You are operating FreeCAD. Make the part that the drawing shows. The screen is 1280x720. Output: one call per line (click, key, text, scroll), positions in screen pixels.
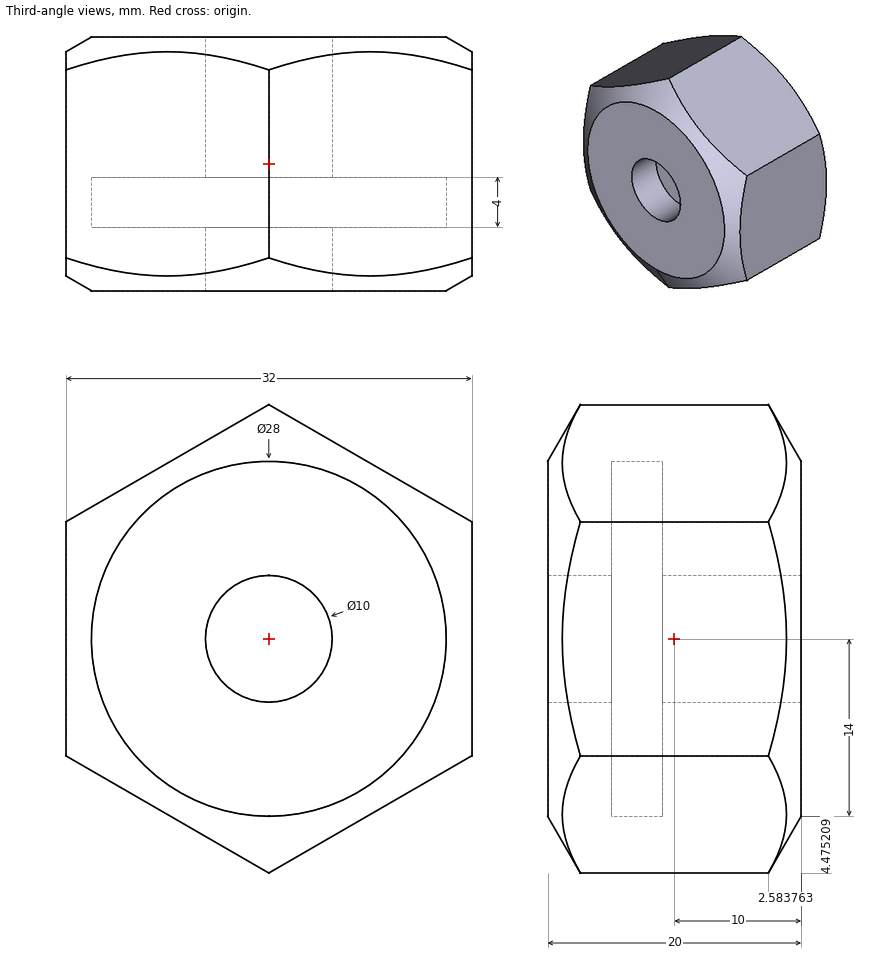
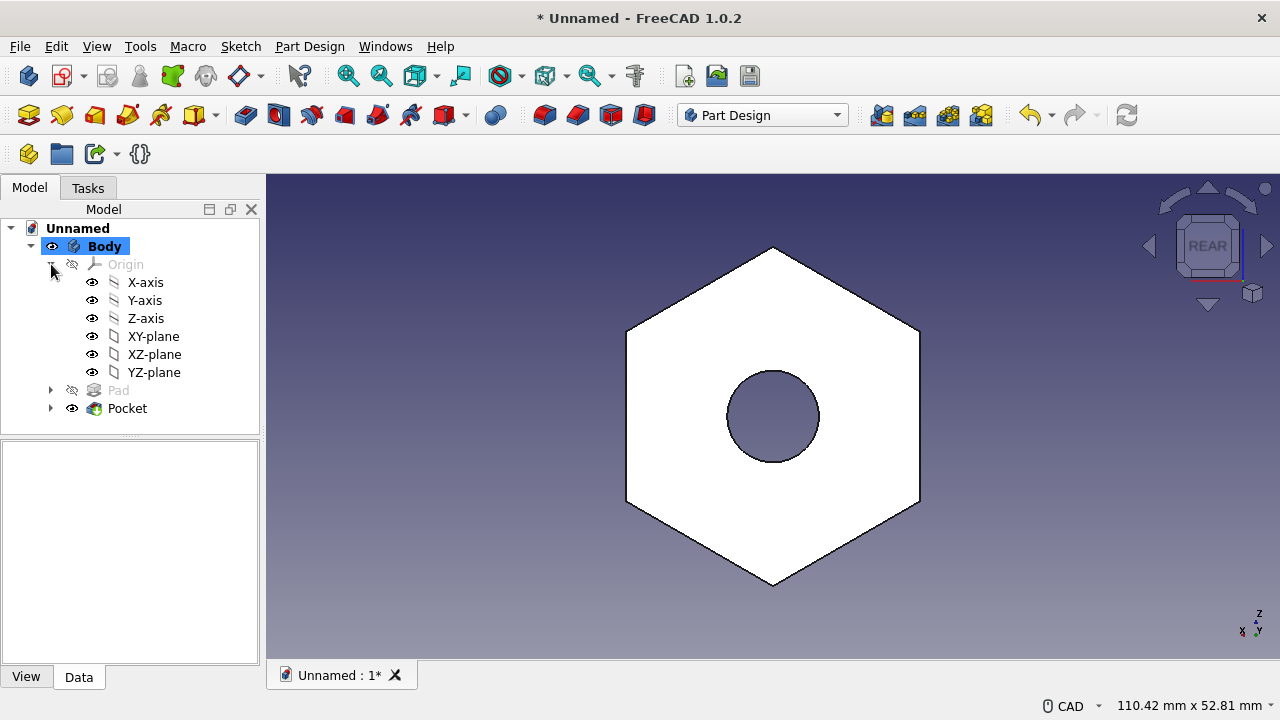
click(137, 354)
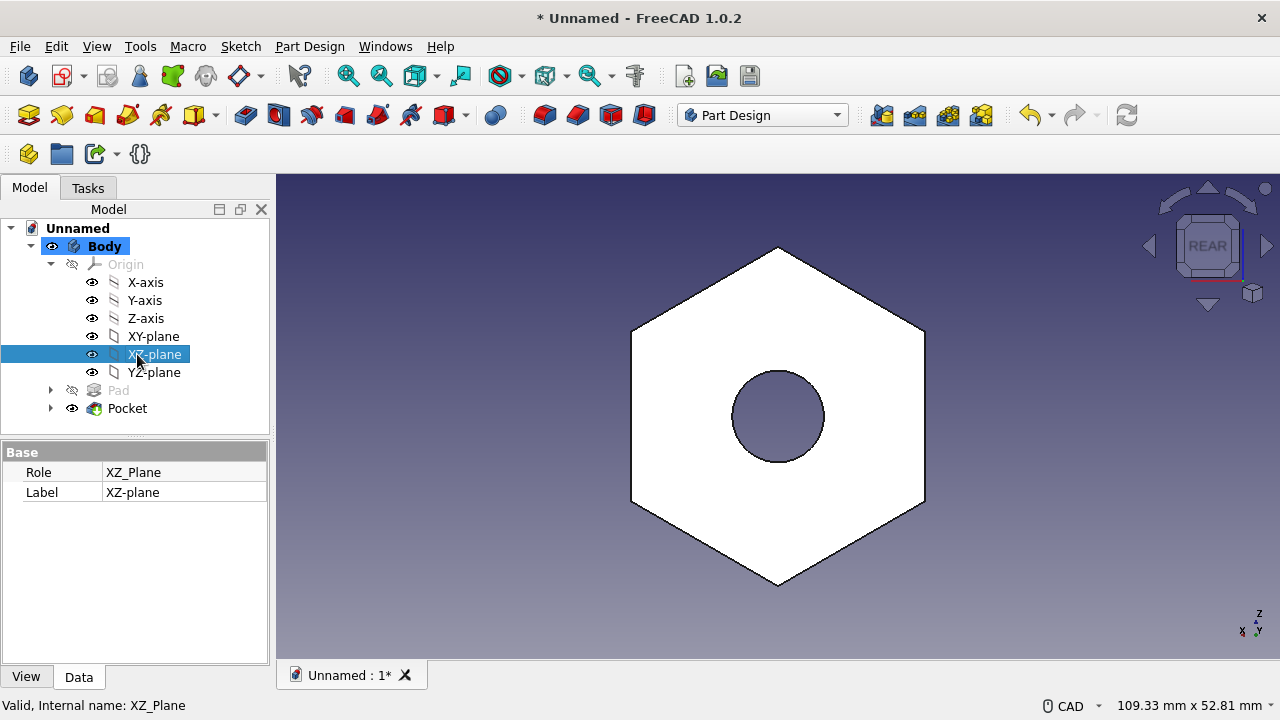
click(238, 76)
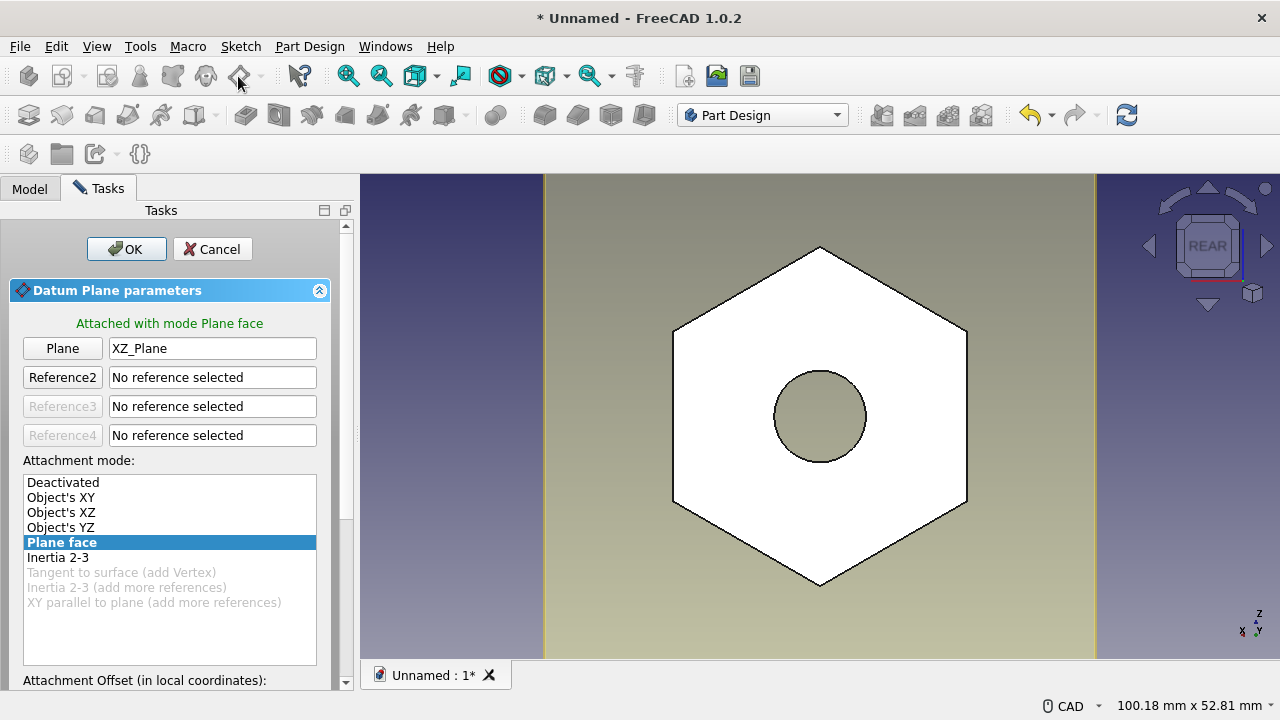
scroll(346, 455, down, 3)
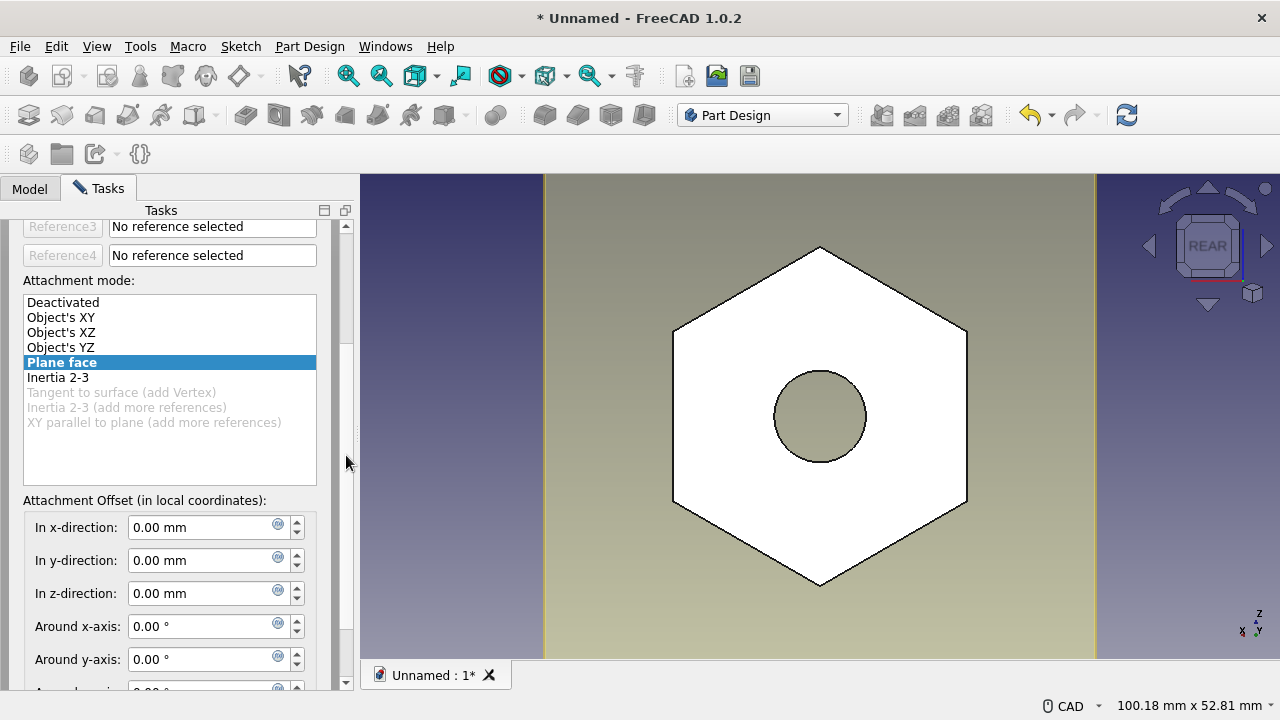
triple_click(210, 594)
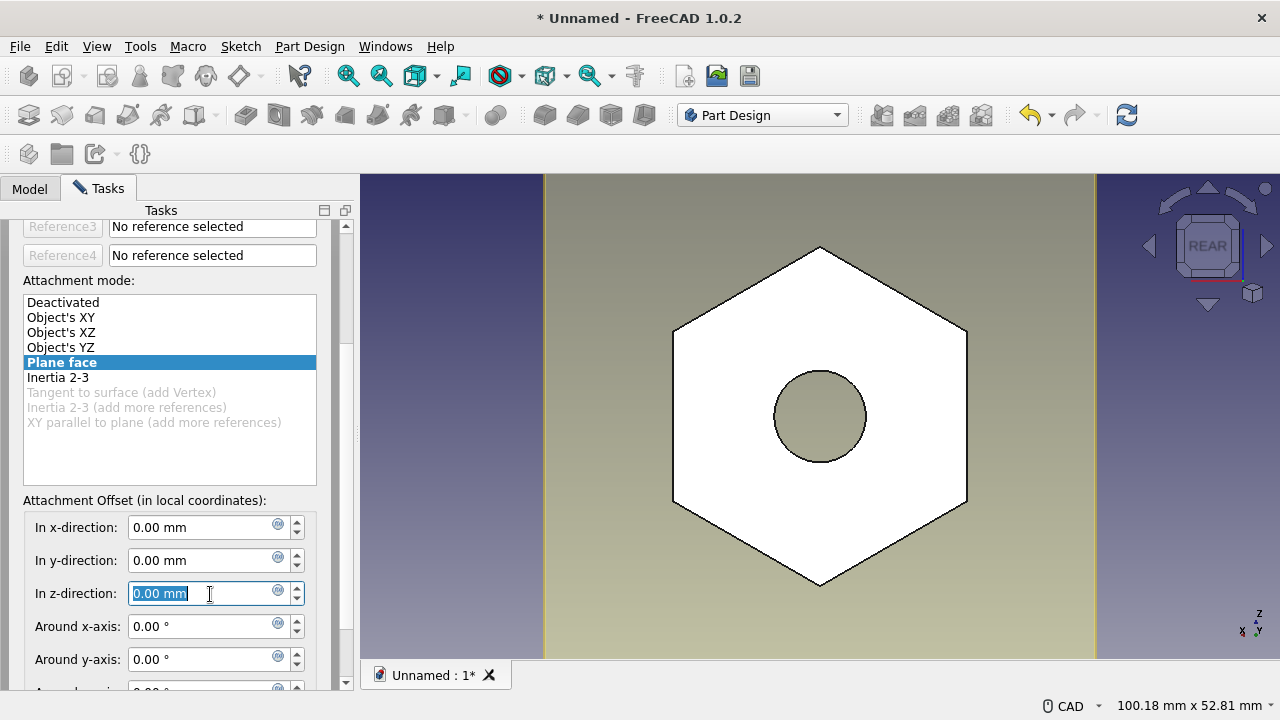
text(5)
key(Tab)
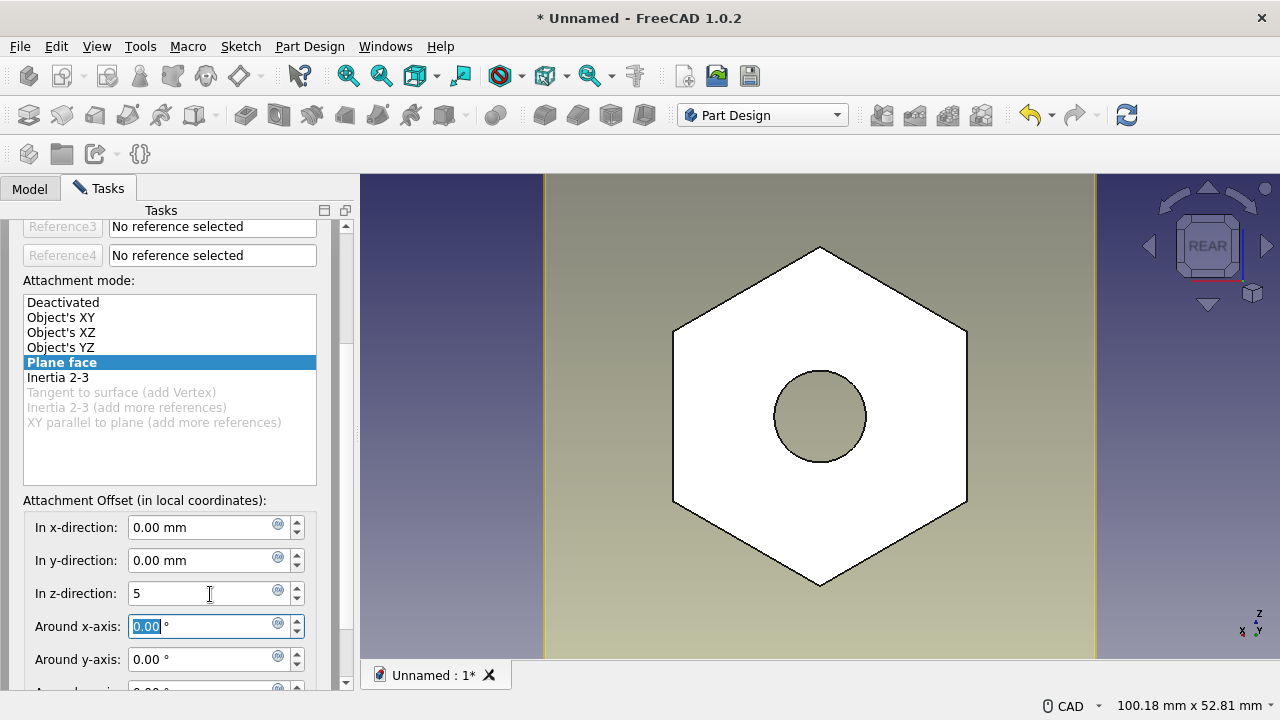
scroll(346, 455, up, 4)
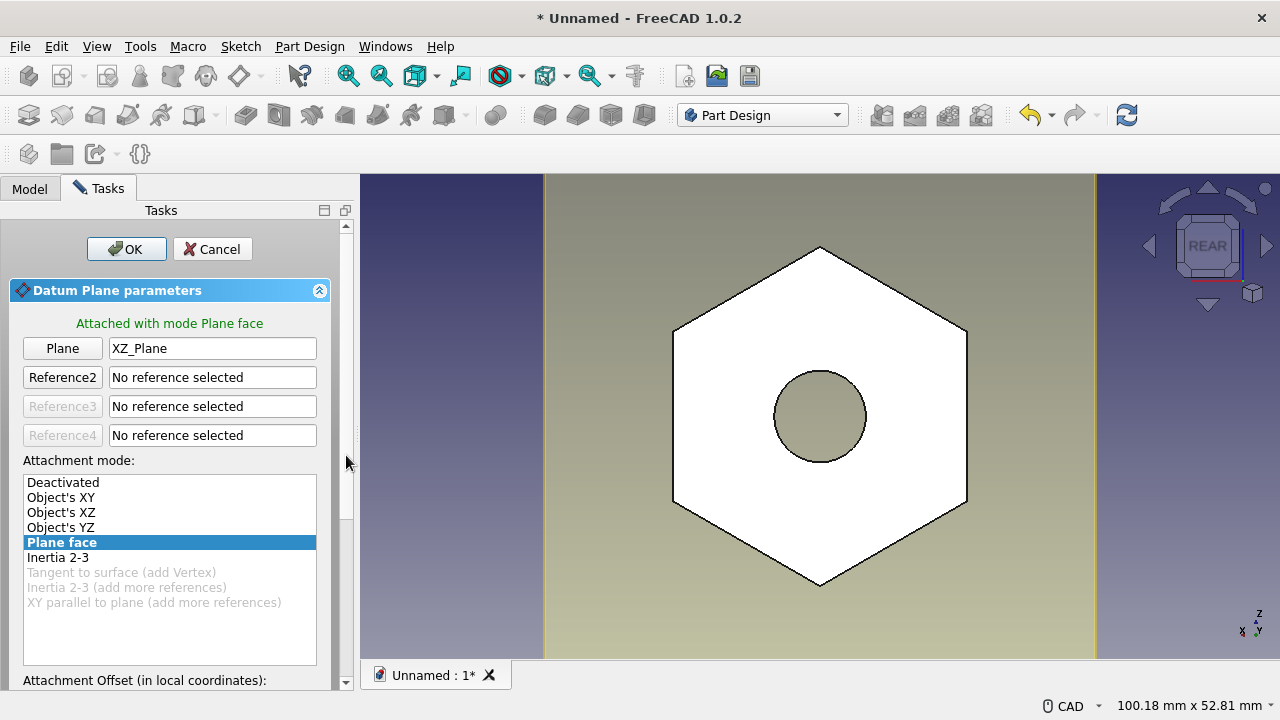
click(127, 249)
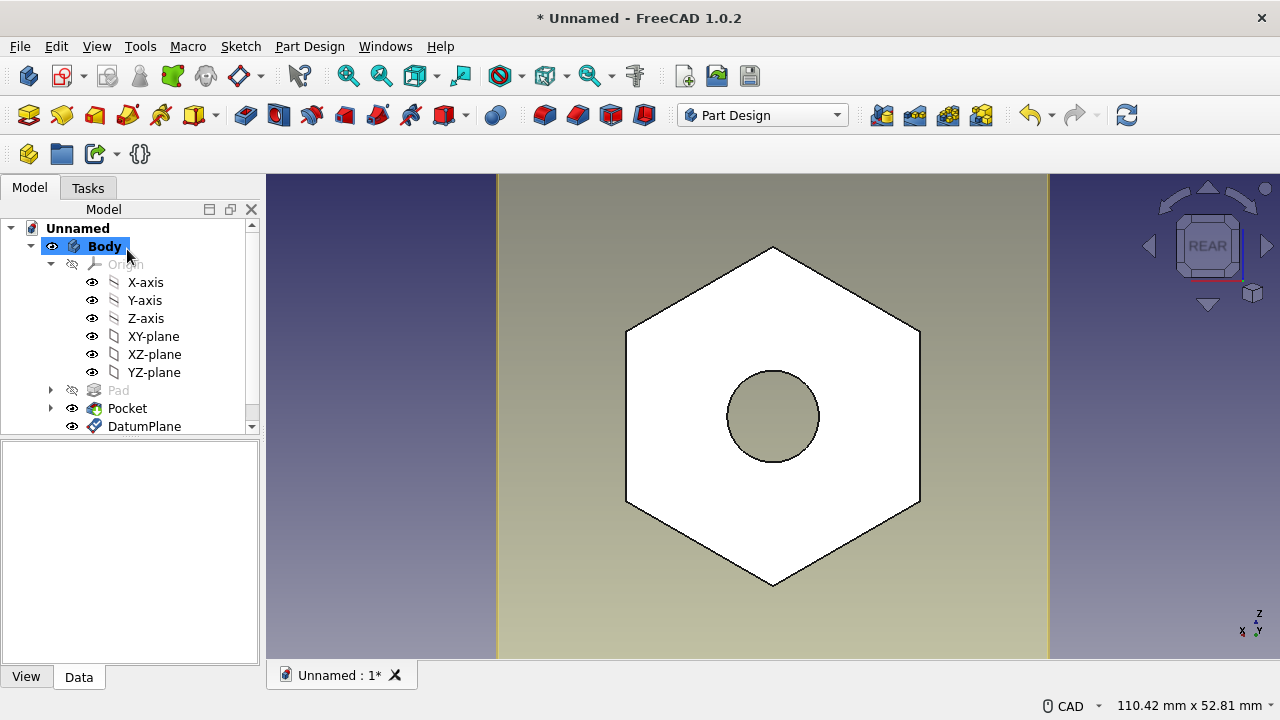
click(117, 426)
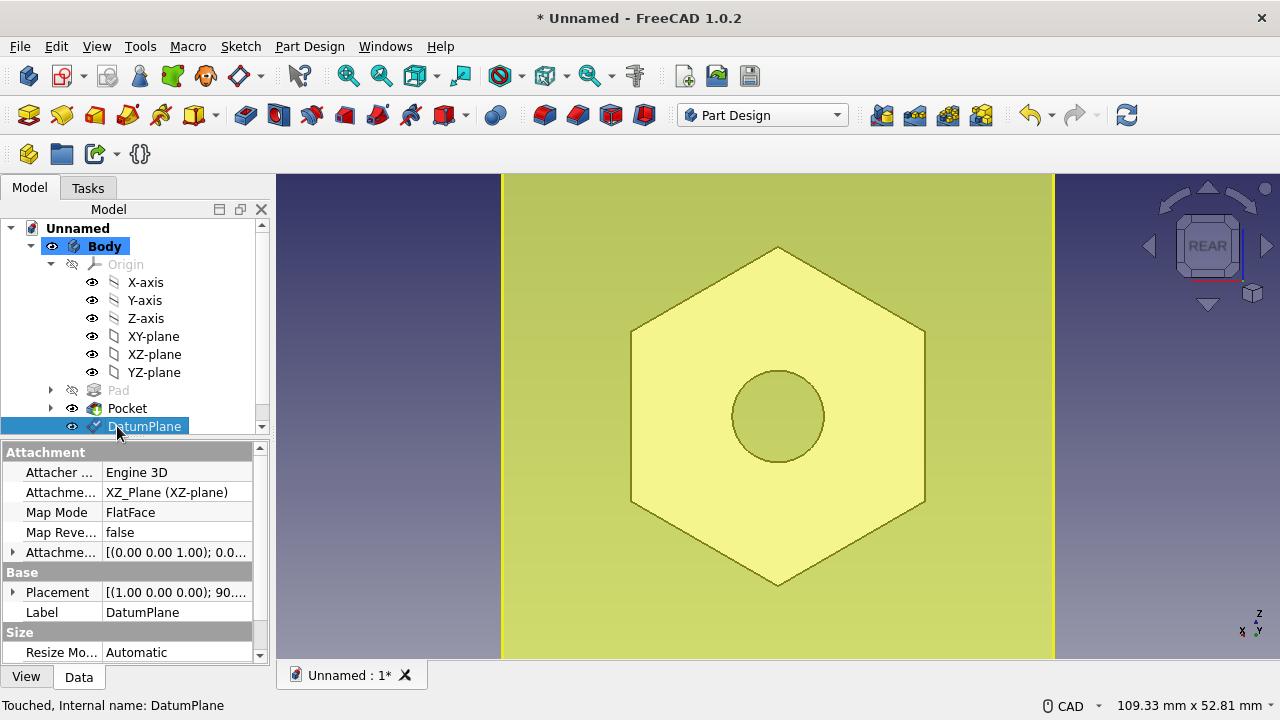
click(62, 76)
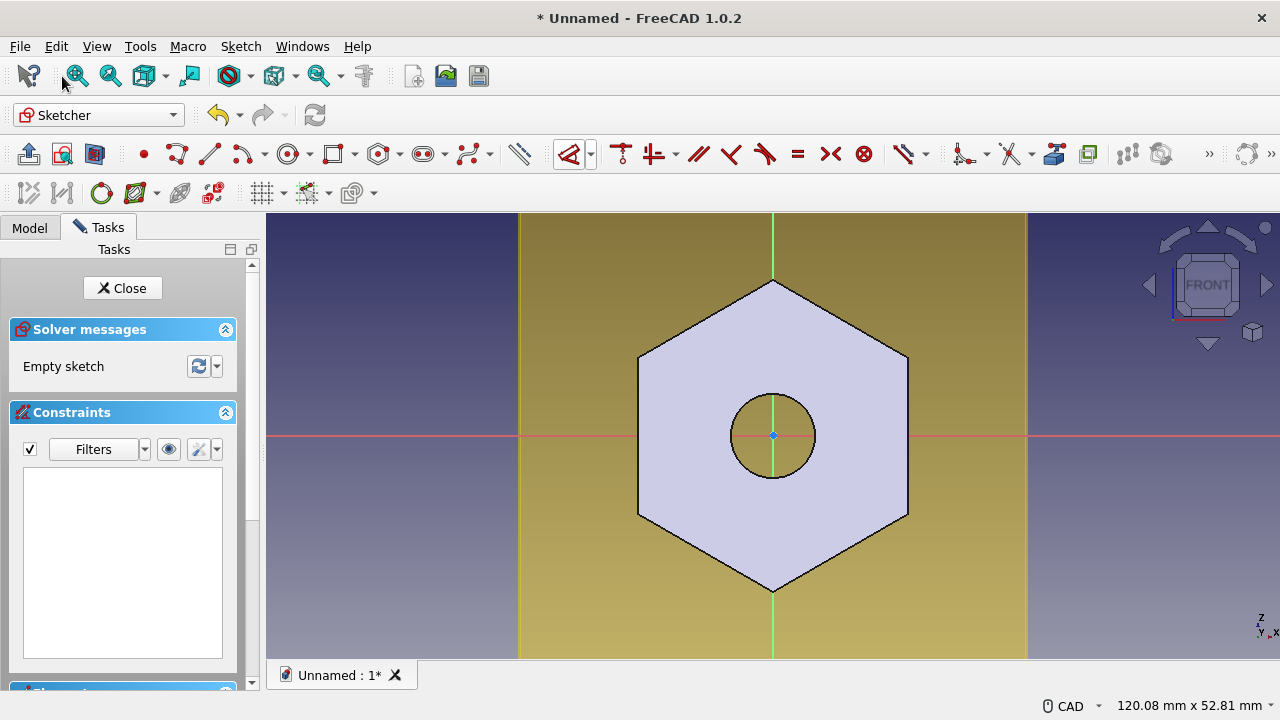
click(95, 154)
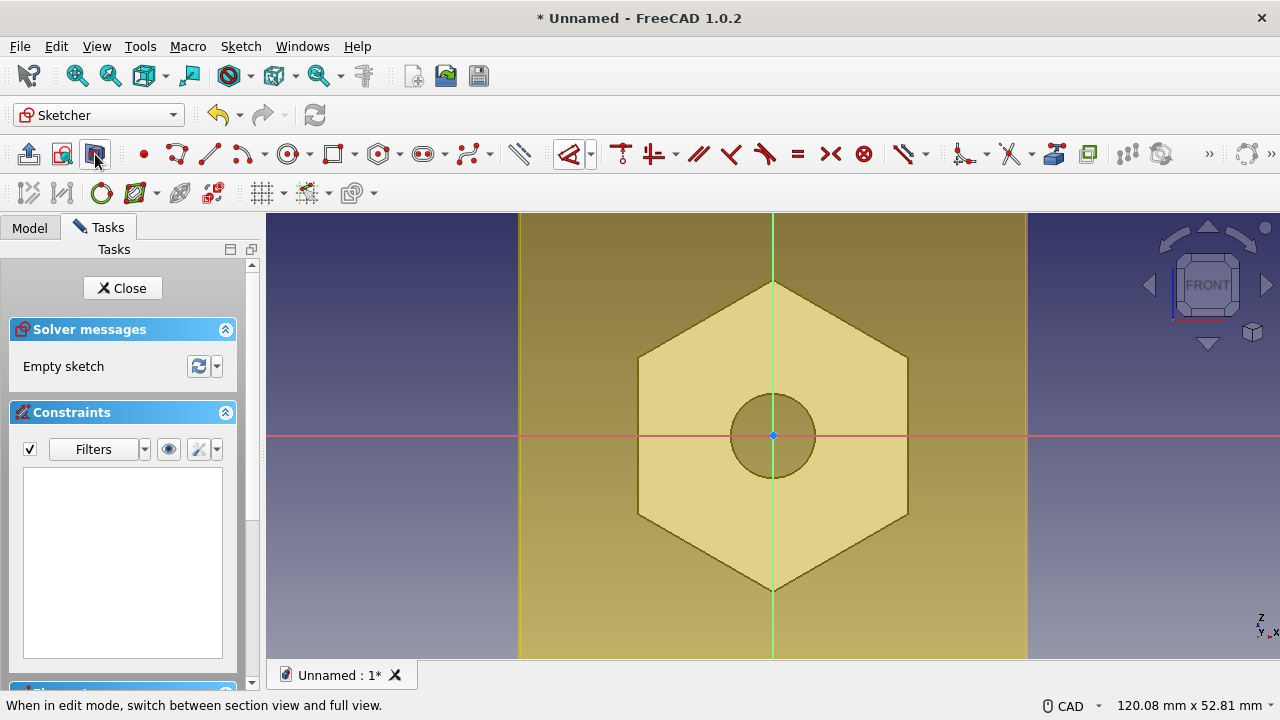
key(g)
key(c)